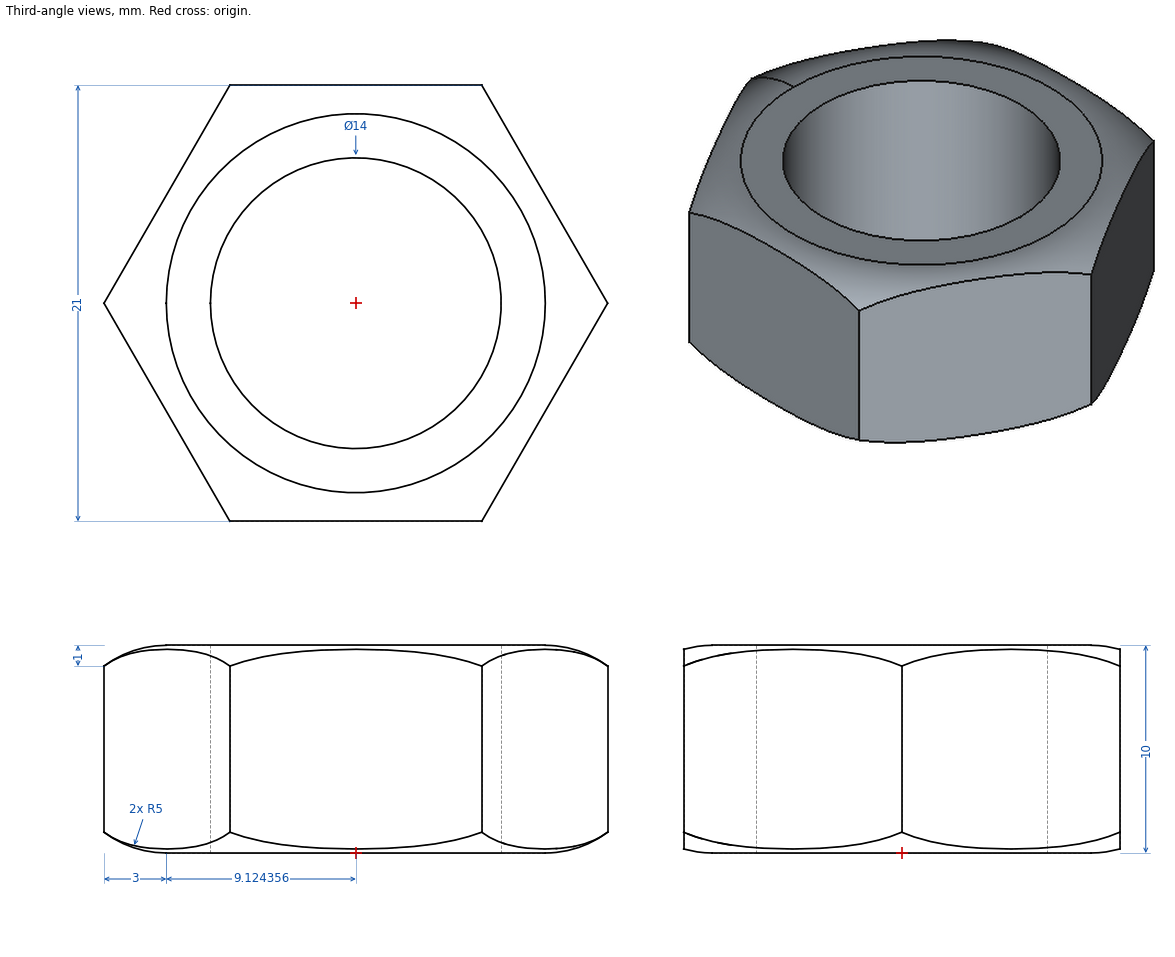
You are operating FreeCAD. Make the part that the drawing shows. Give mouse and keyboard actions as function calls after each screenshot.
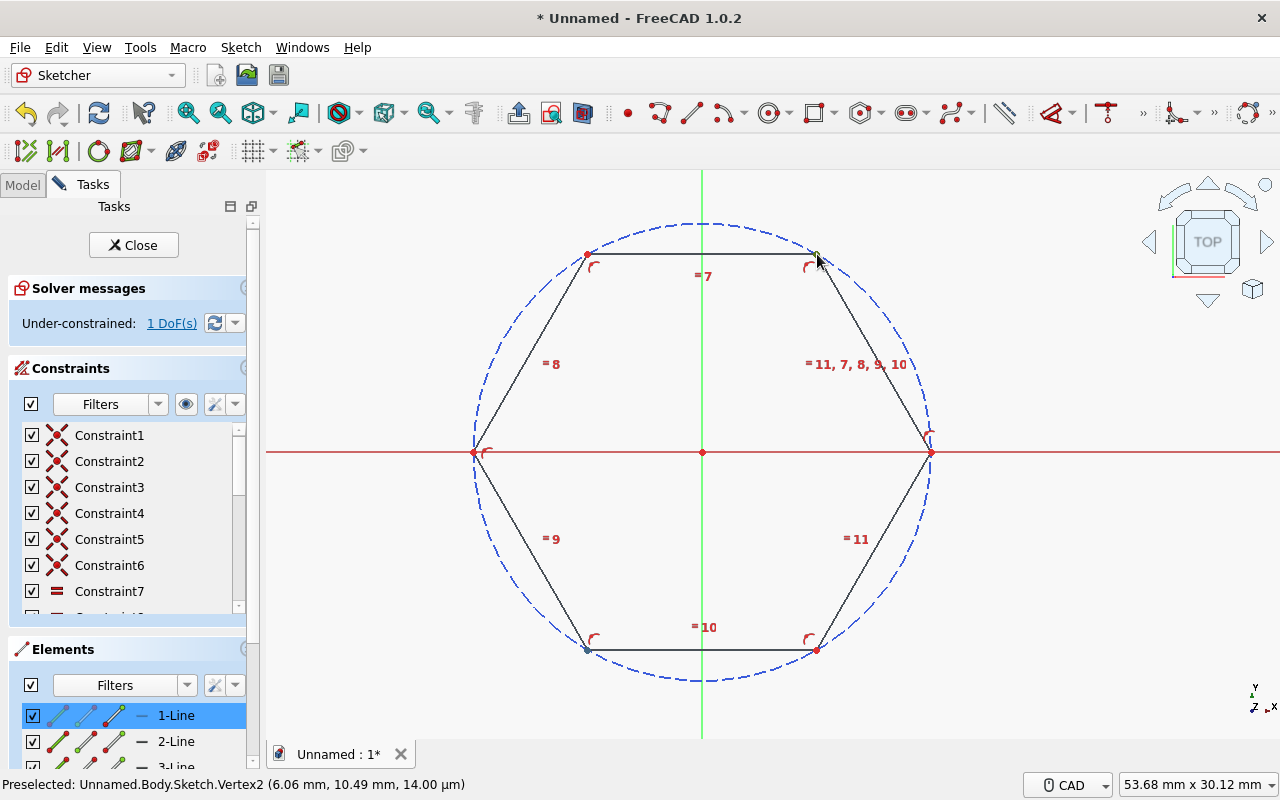
key(i)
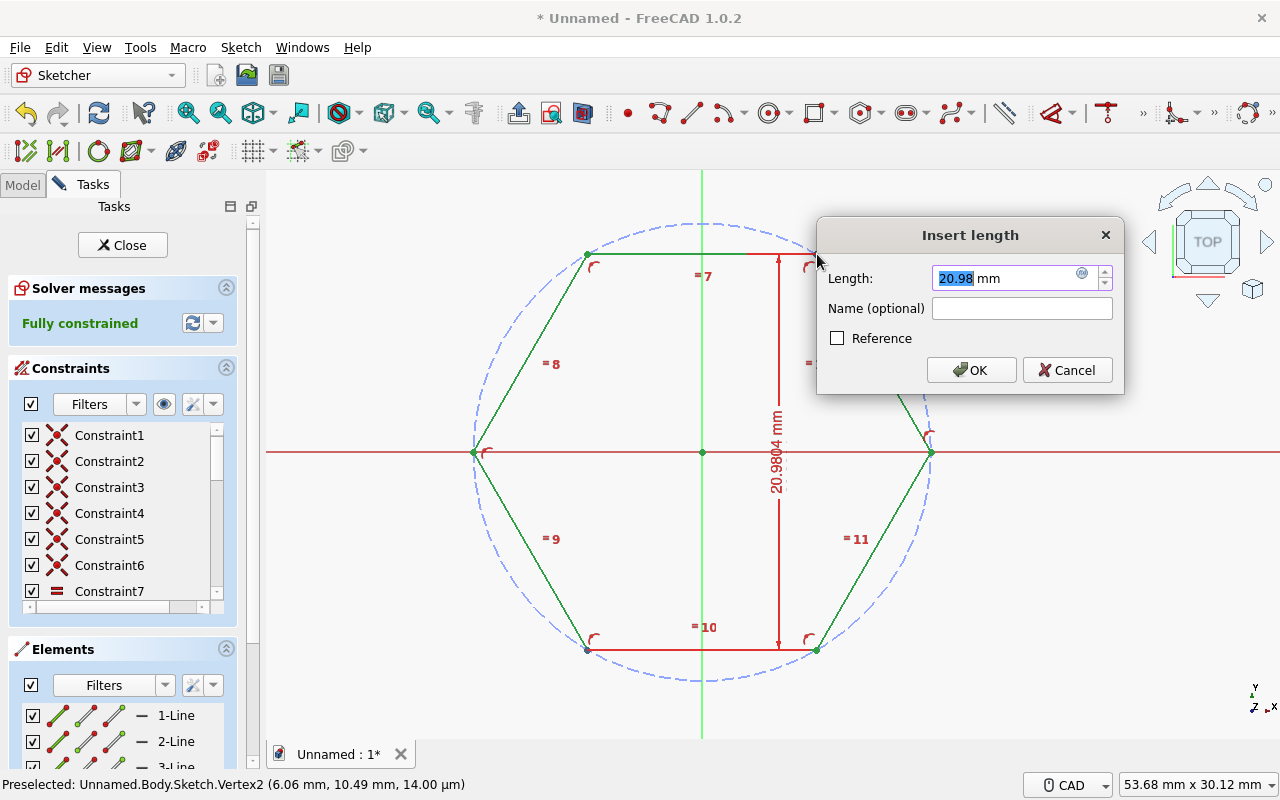
text(21)
key(Return)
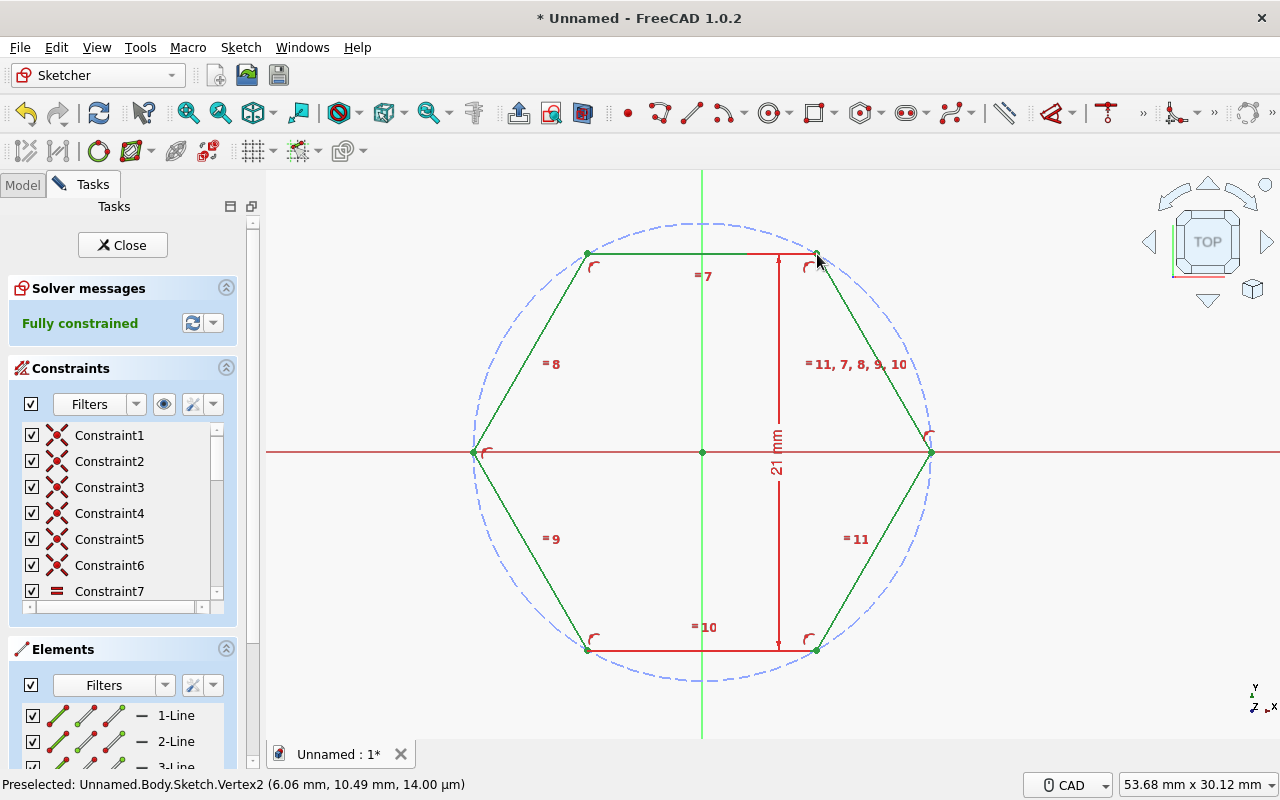
click(123, 245)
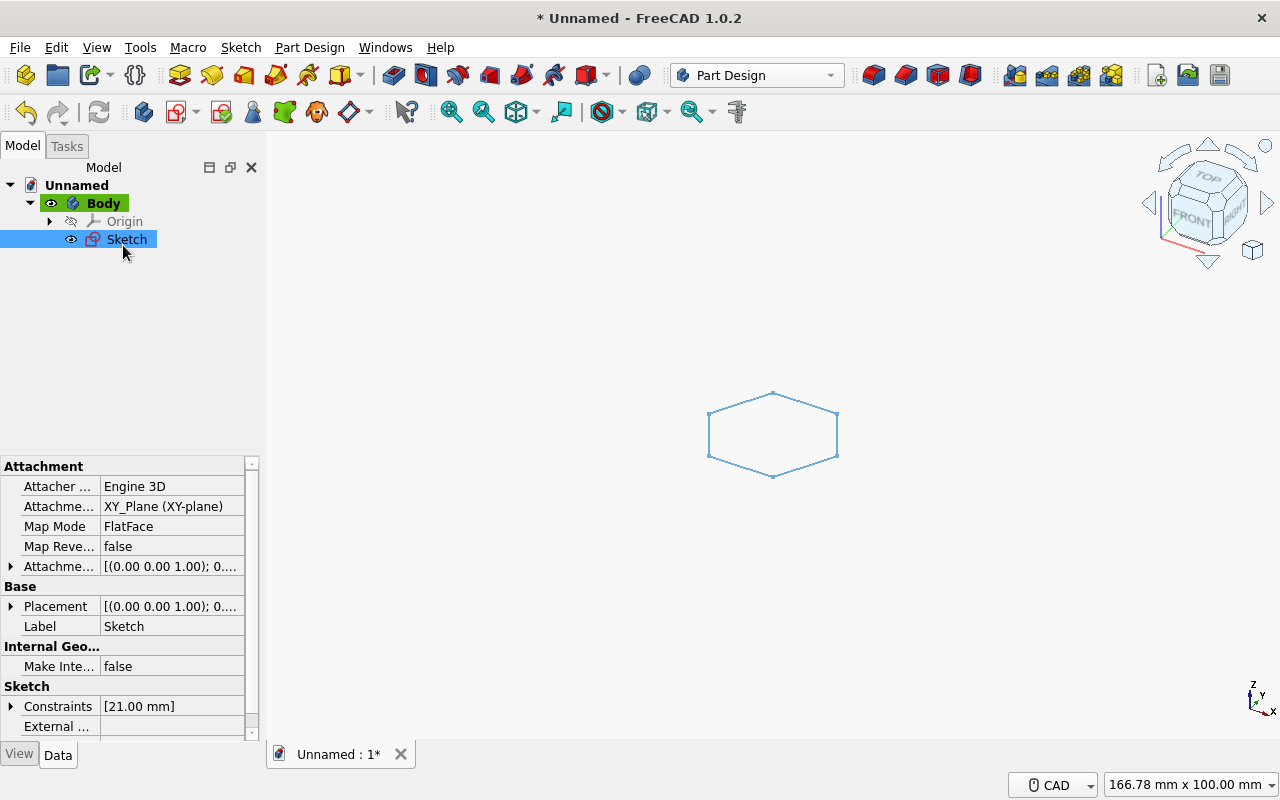
click(180, 76)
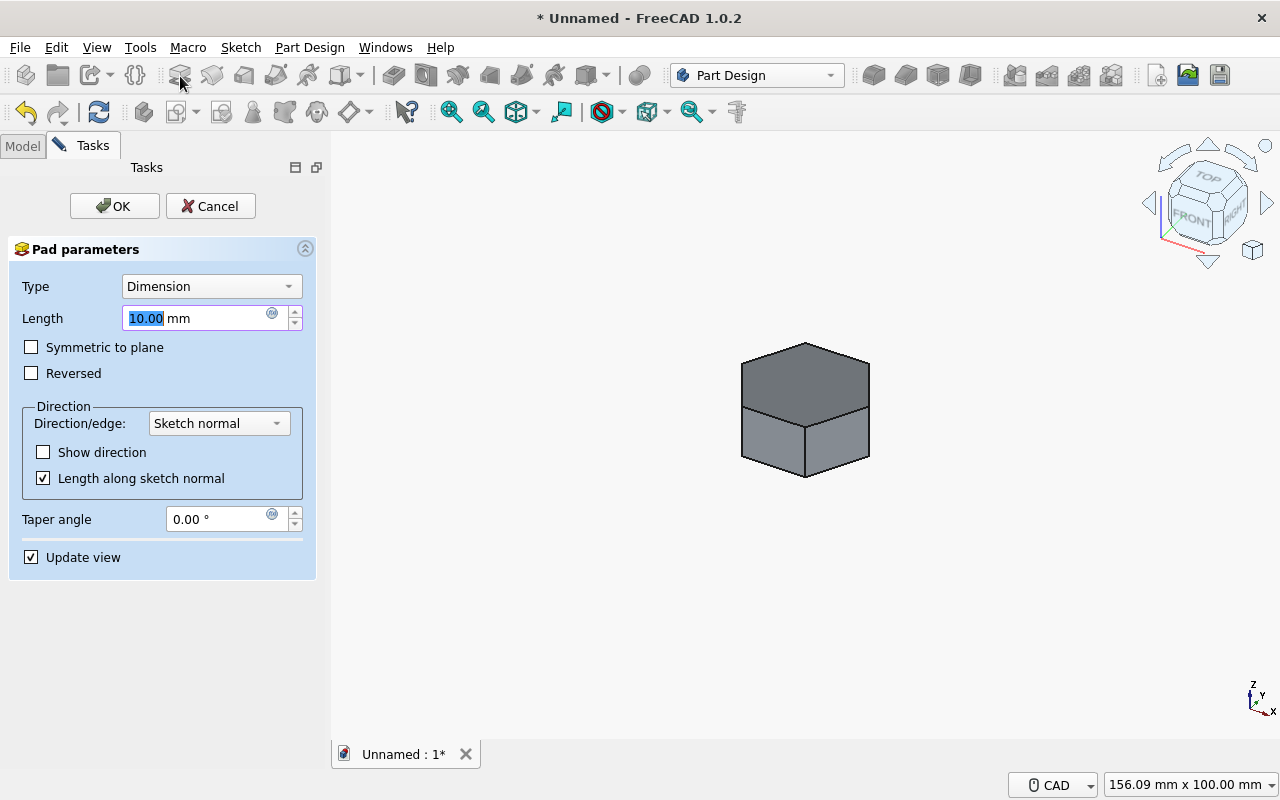
text(10)
key(Tab)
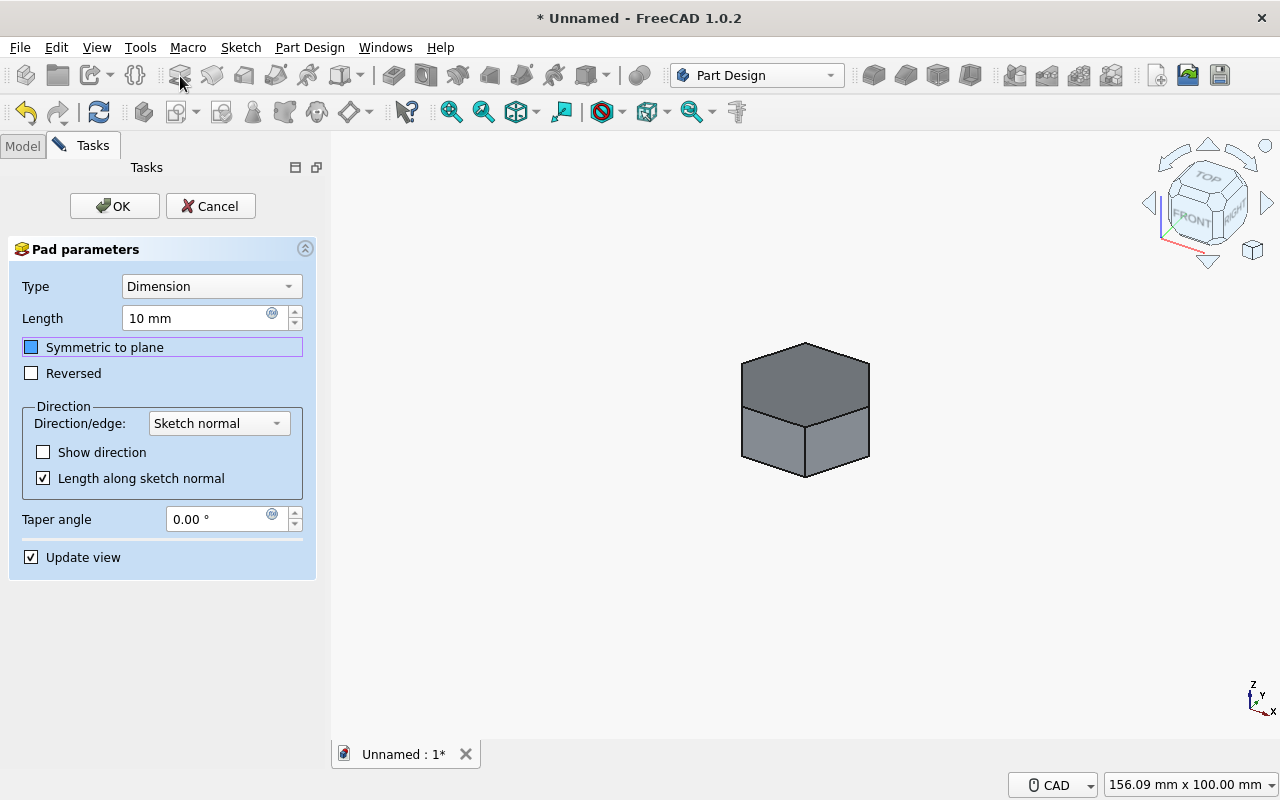
click(115, 206)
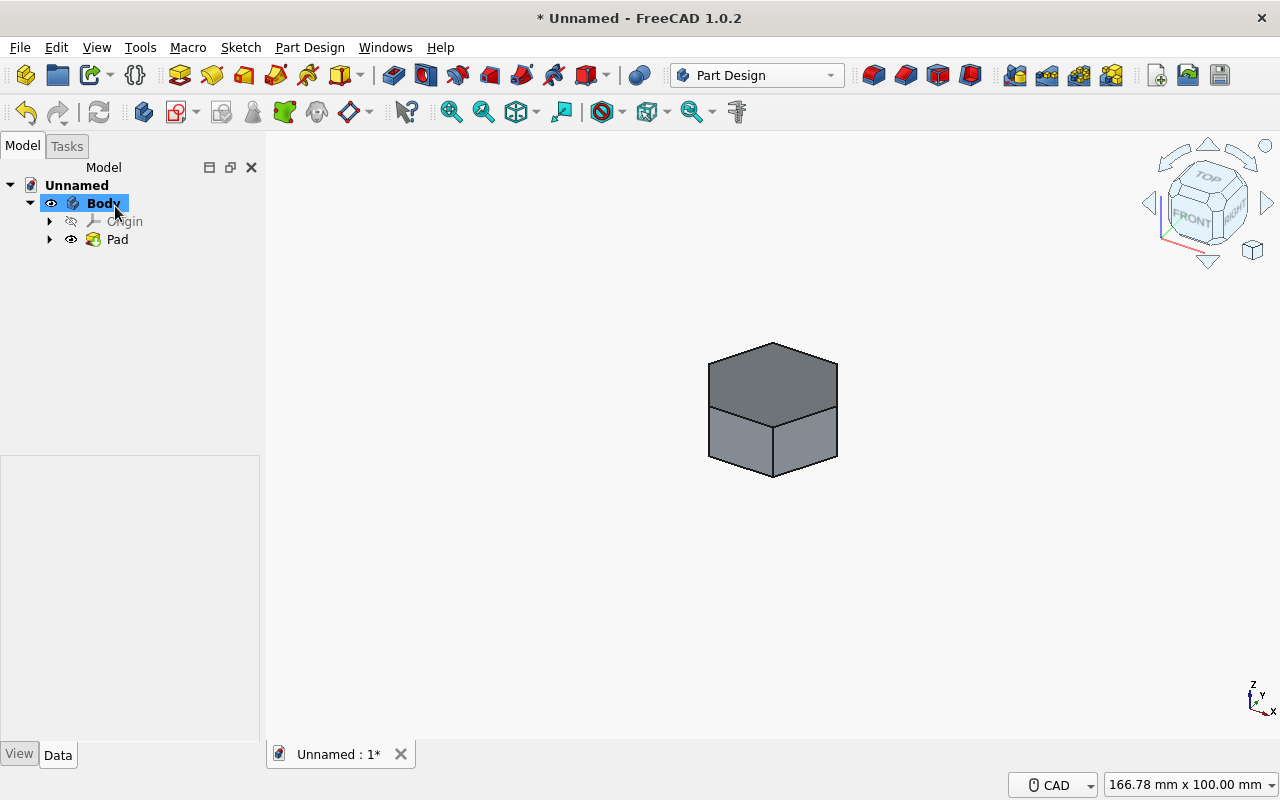
click(452, 112)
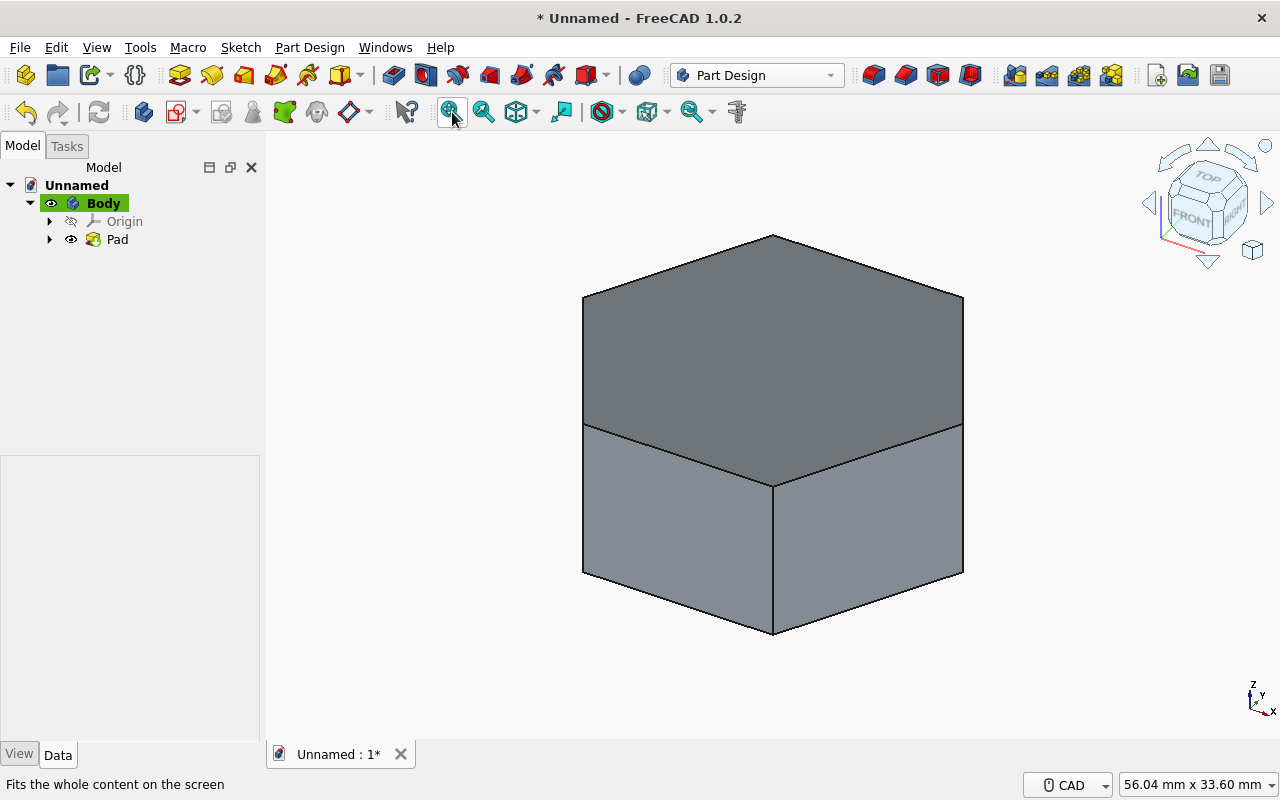
click(176, 112)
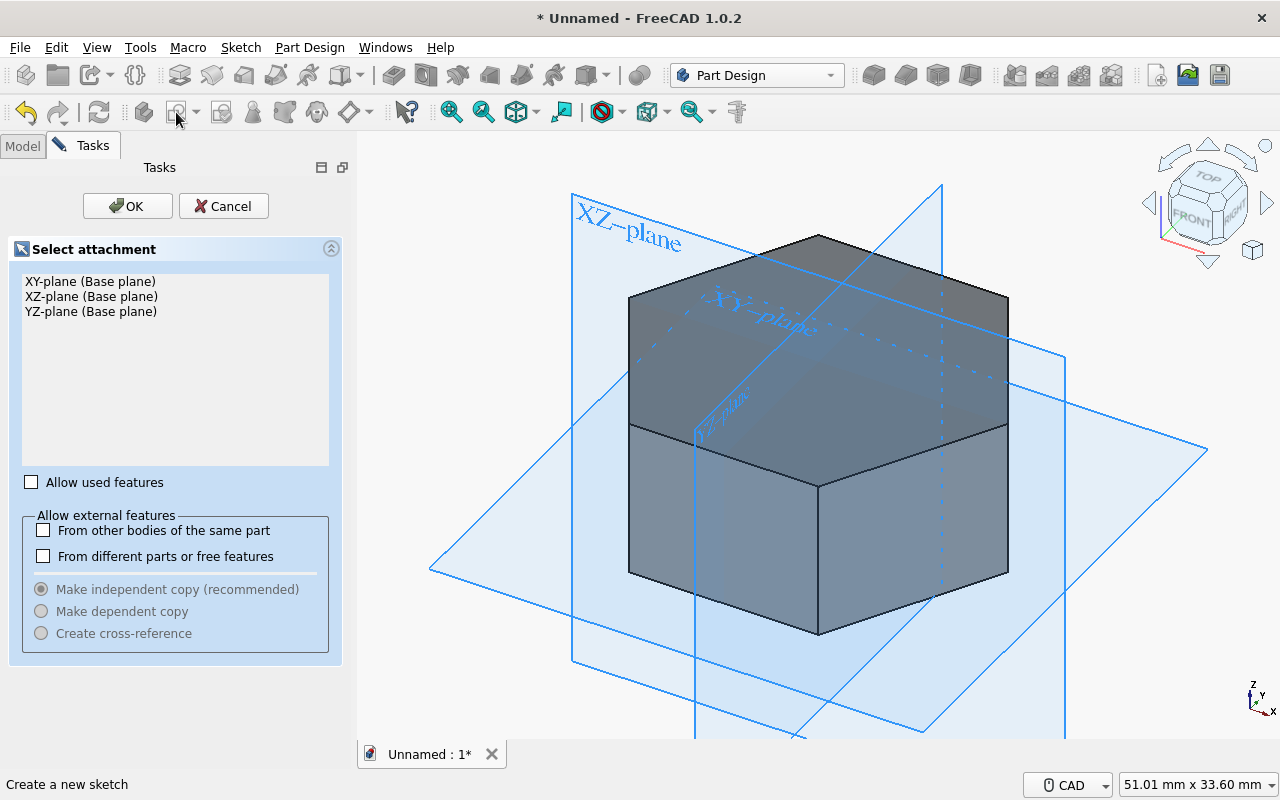
click(82, 296)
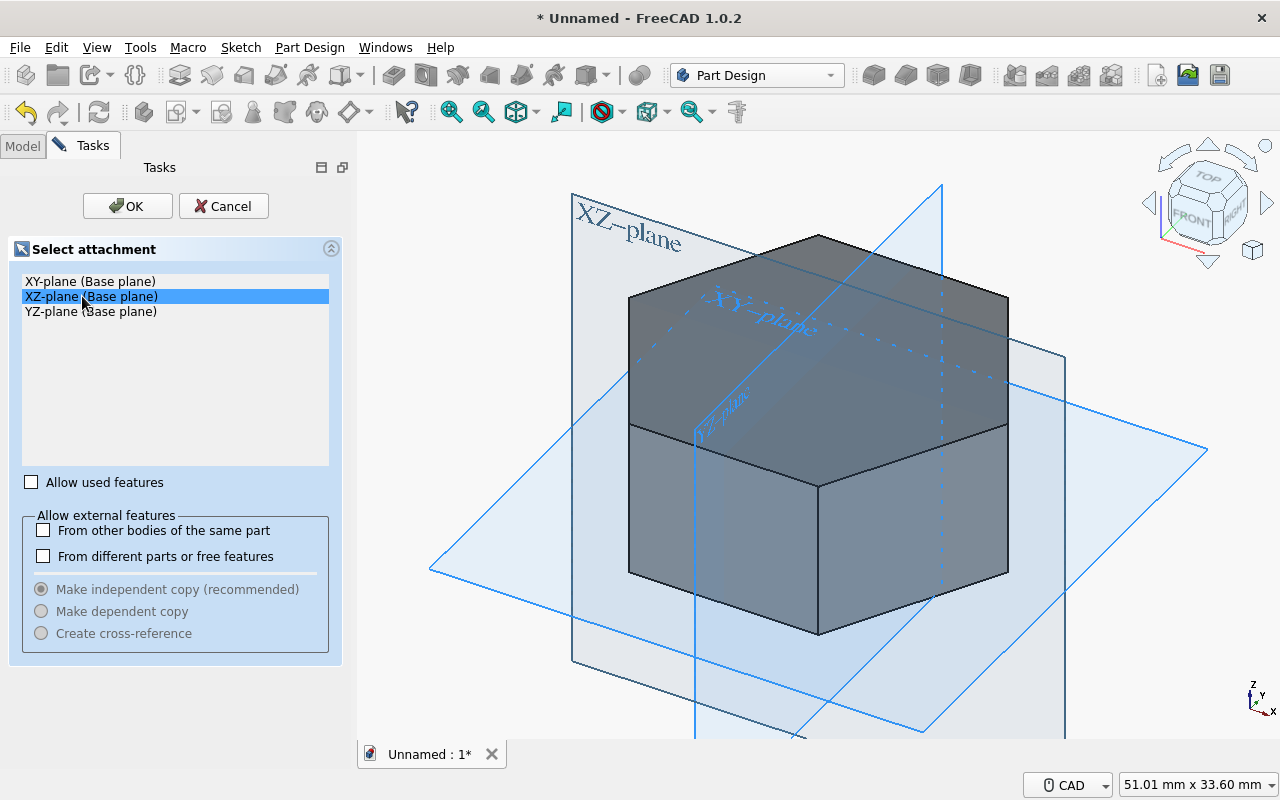
click(128, 206)